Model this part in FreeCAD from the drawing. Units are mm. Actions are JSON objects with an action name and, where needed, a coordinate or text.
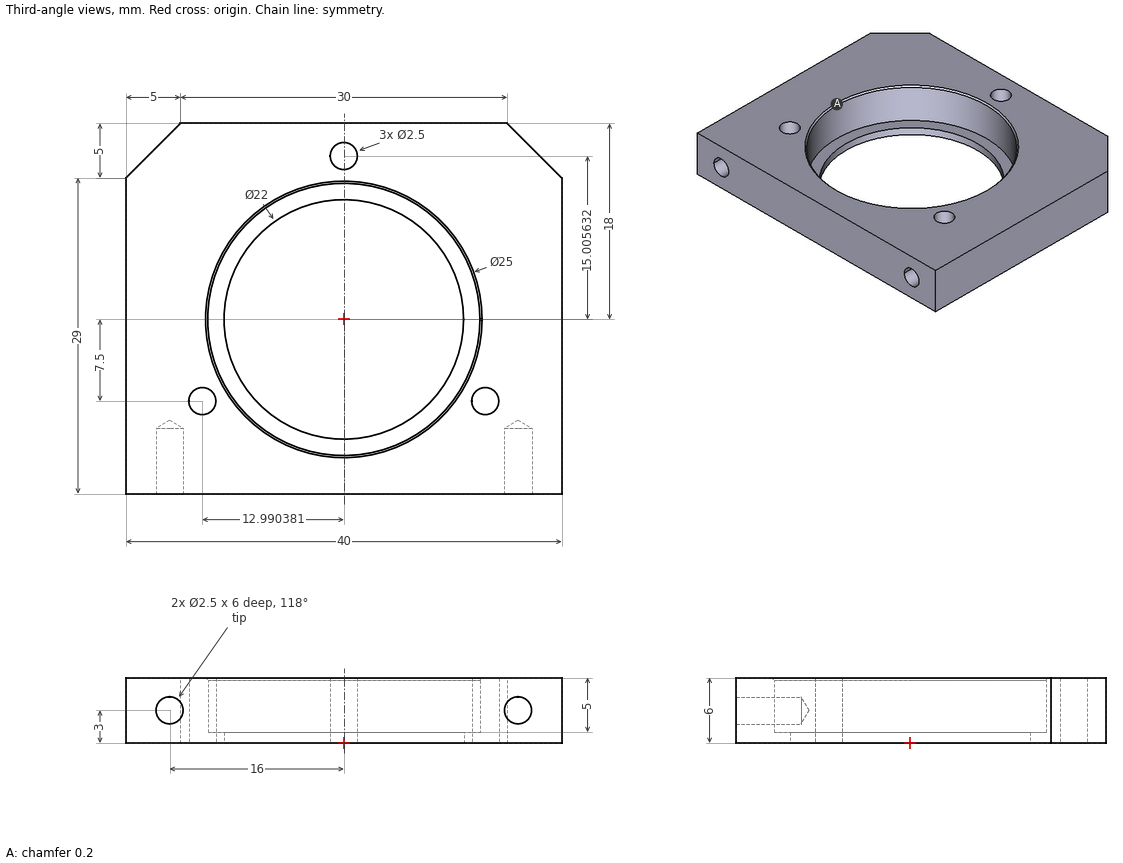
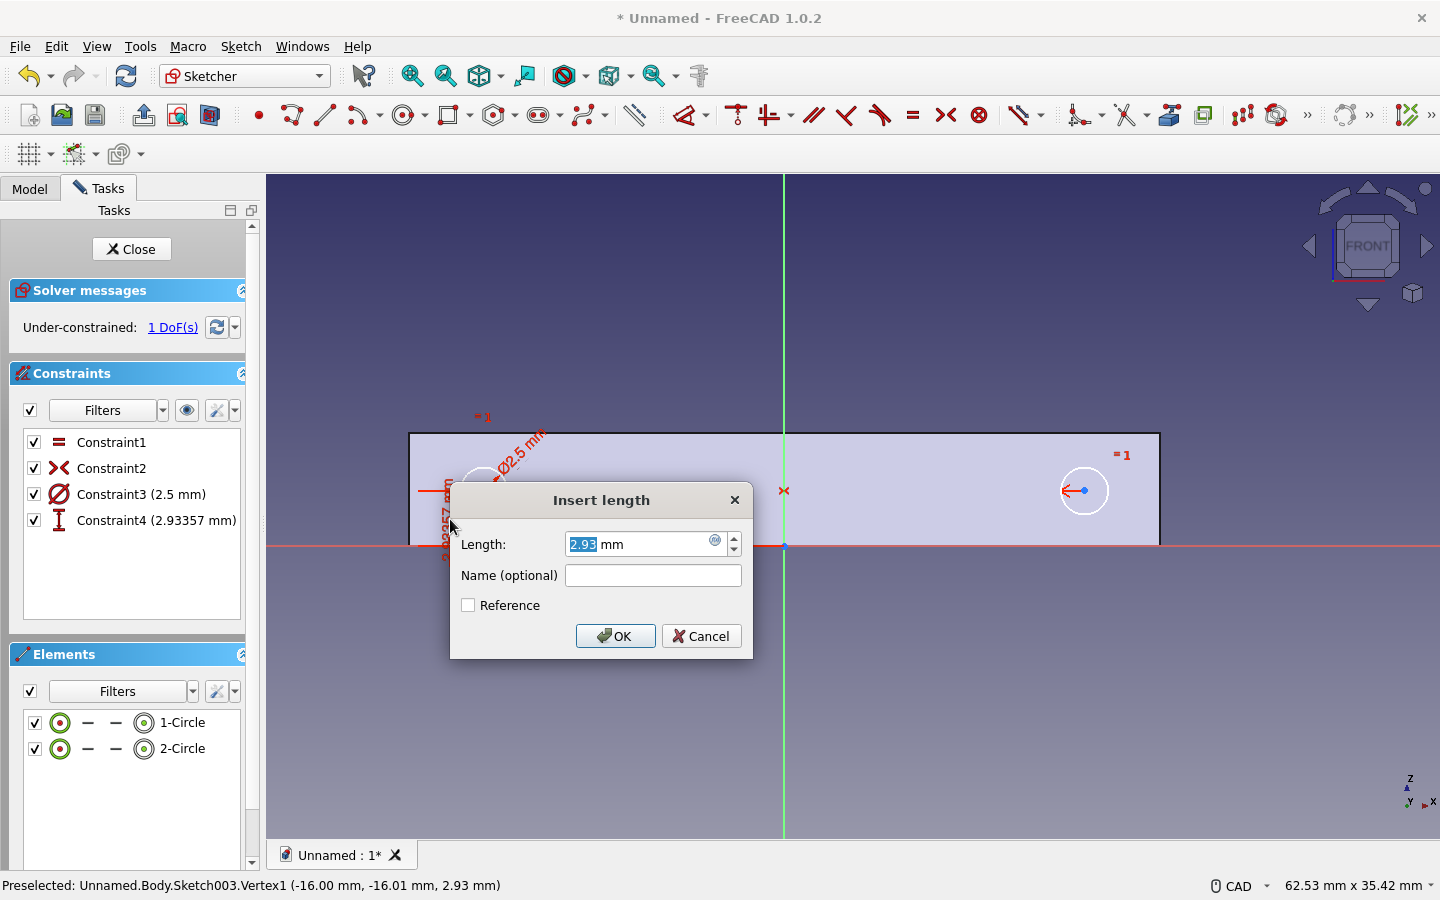
{"action": "type", "text": "3"}
{"action": "key", "text": "Return"}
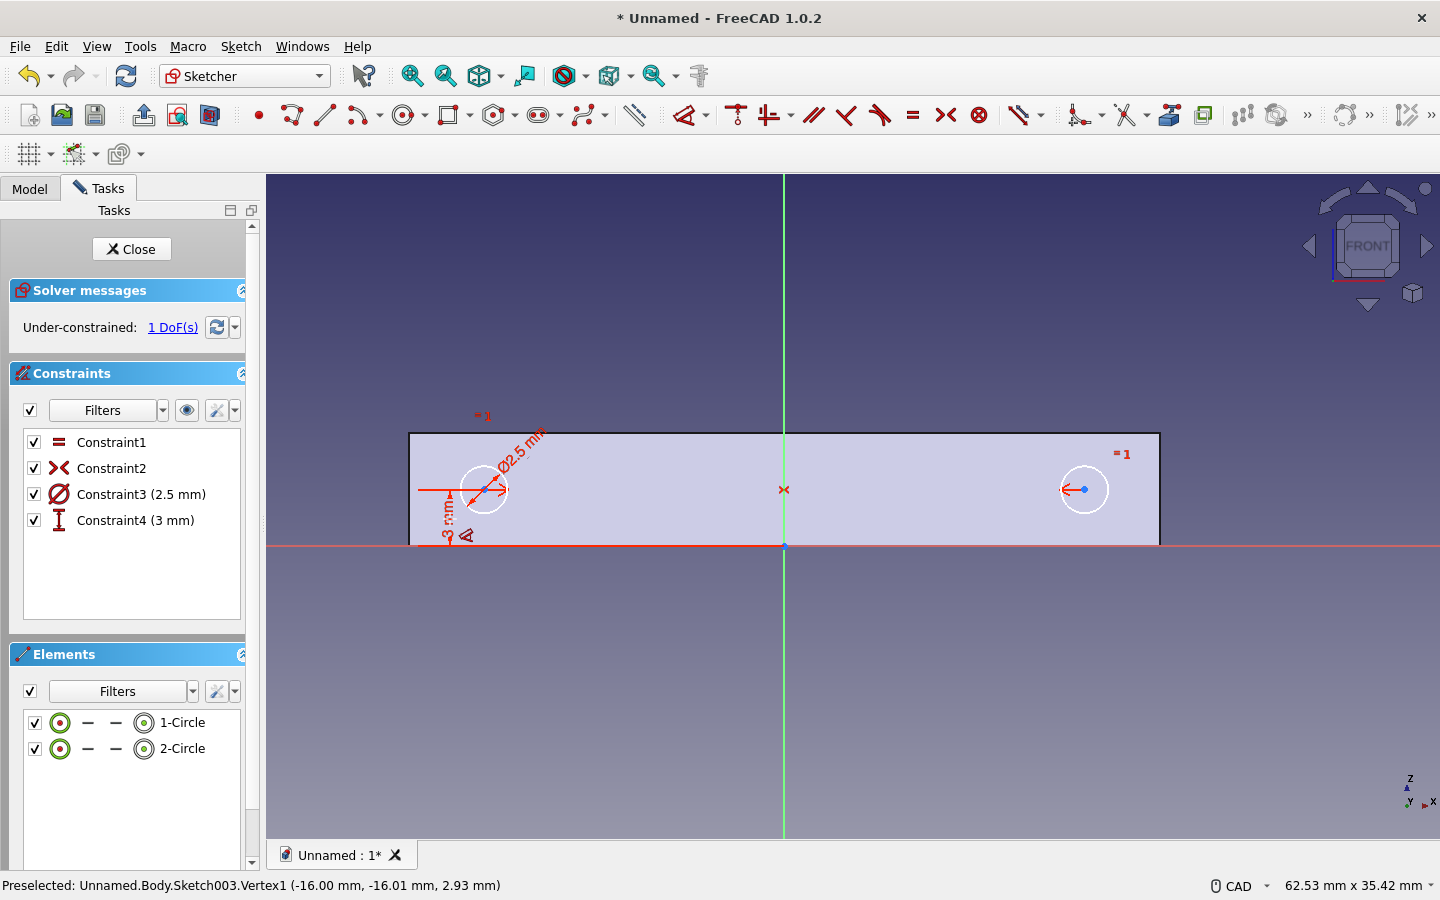
{"action": "left_click", "coordinate": [484, 490]}
{"action": "left_click", "coordinate": [634, 580]}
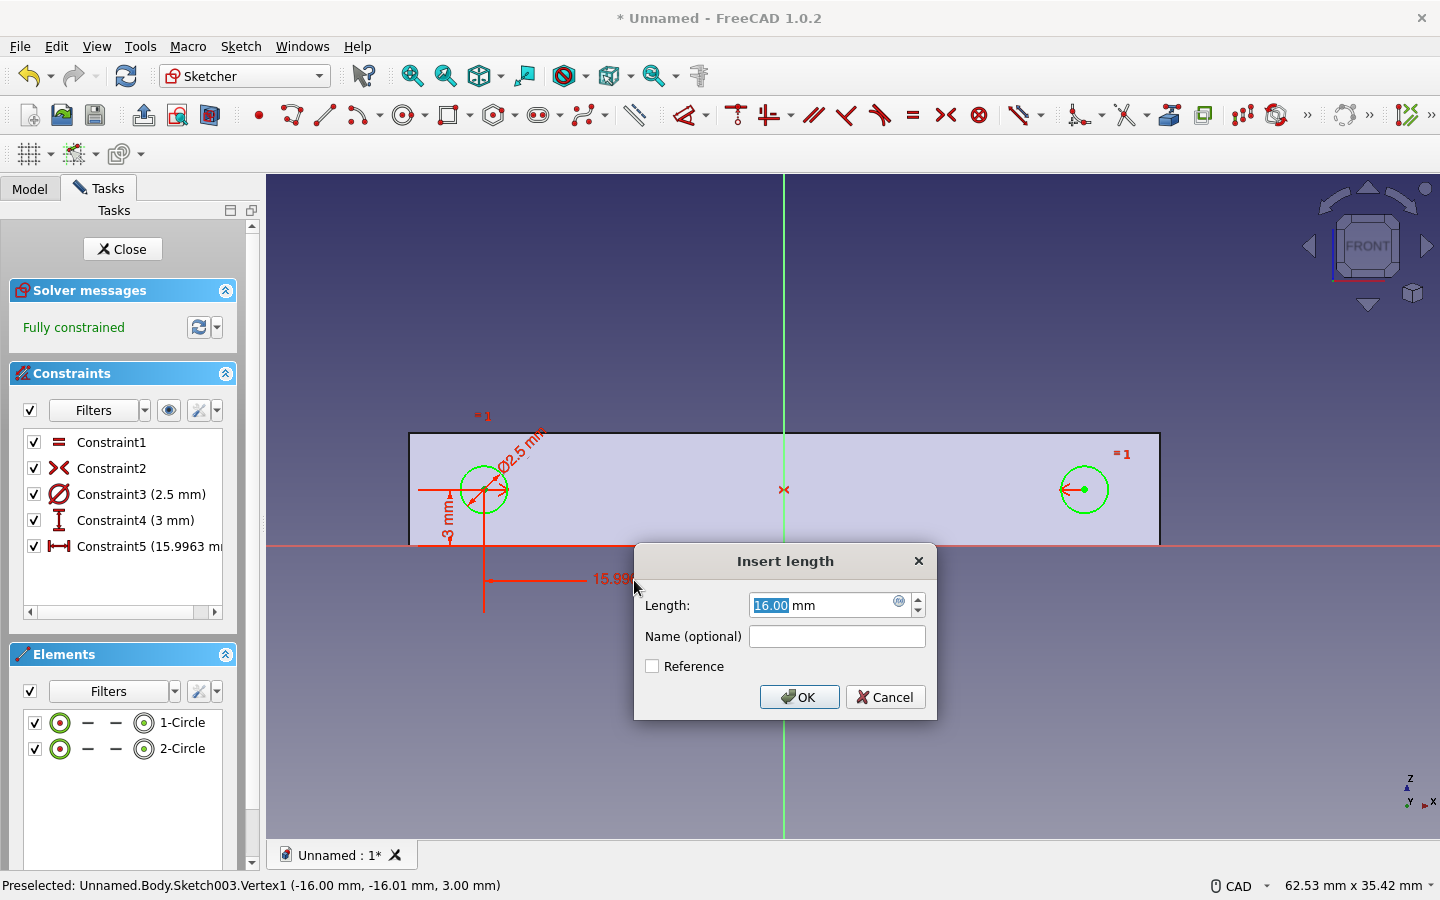
{"action": "type", "text": "16"}
{"action": "key", "text": "Return"}
{"action": "key", "text": "Escape"}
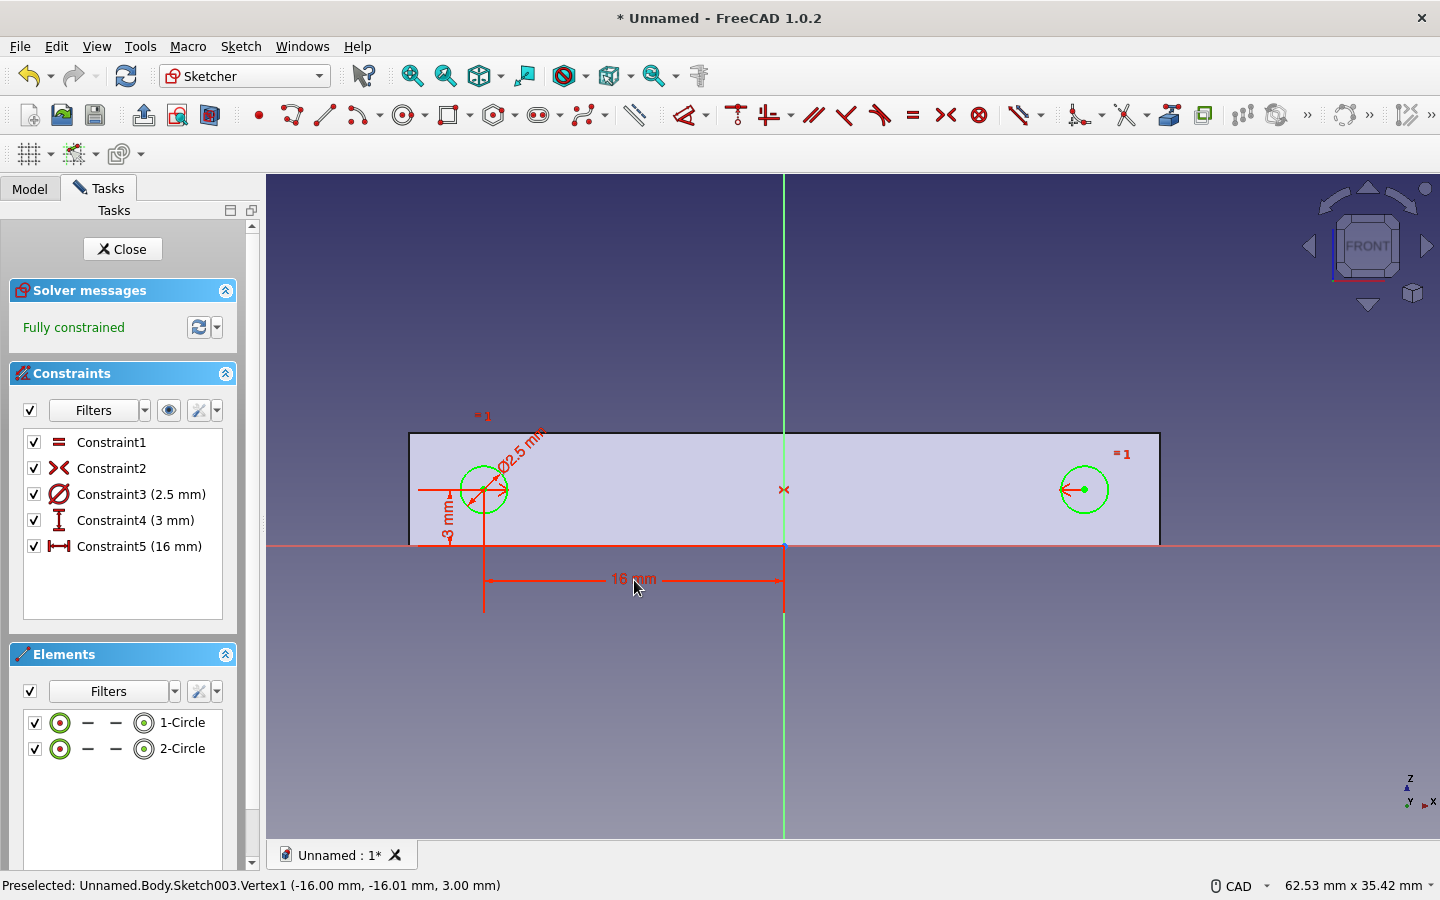
{"action": "left_click", "coordinate": [123, 249]}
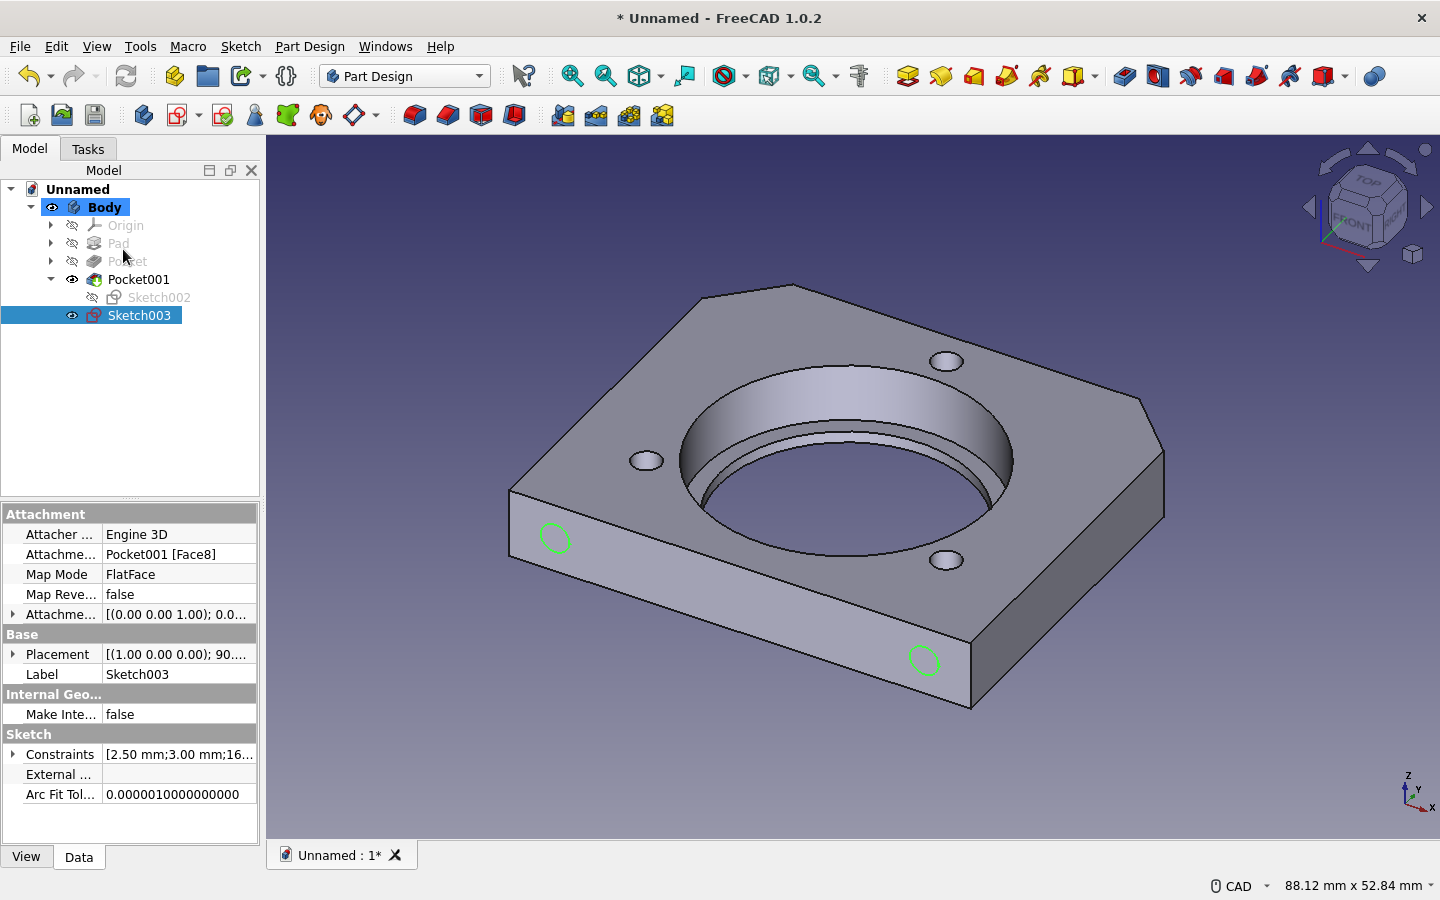
{"action": "left_click", "coordinate": [1158, 76]}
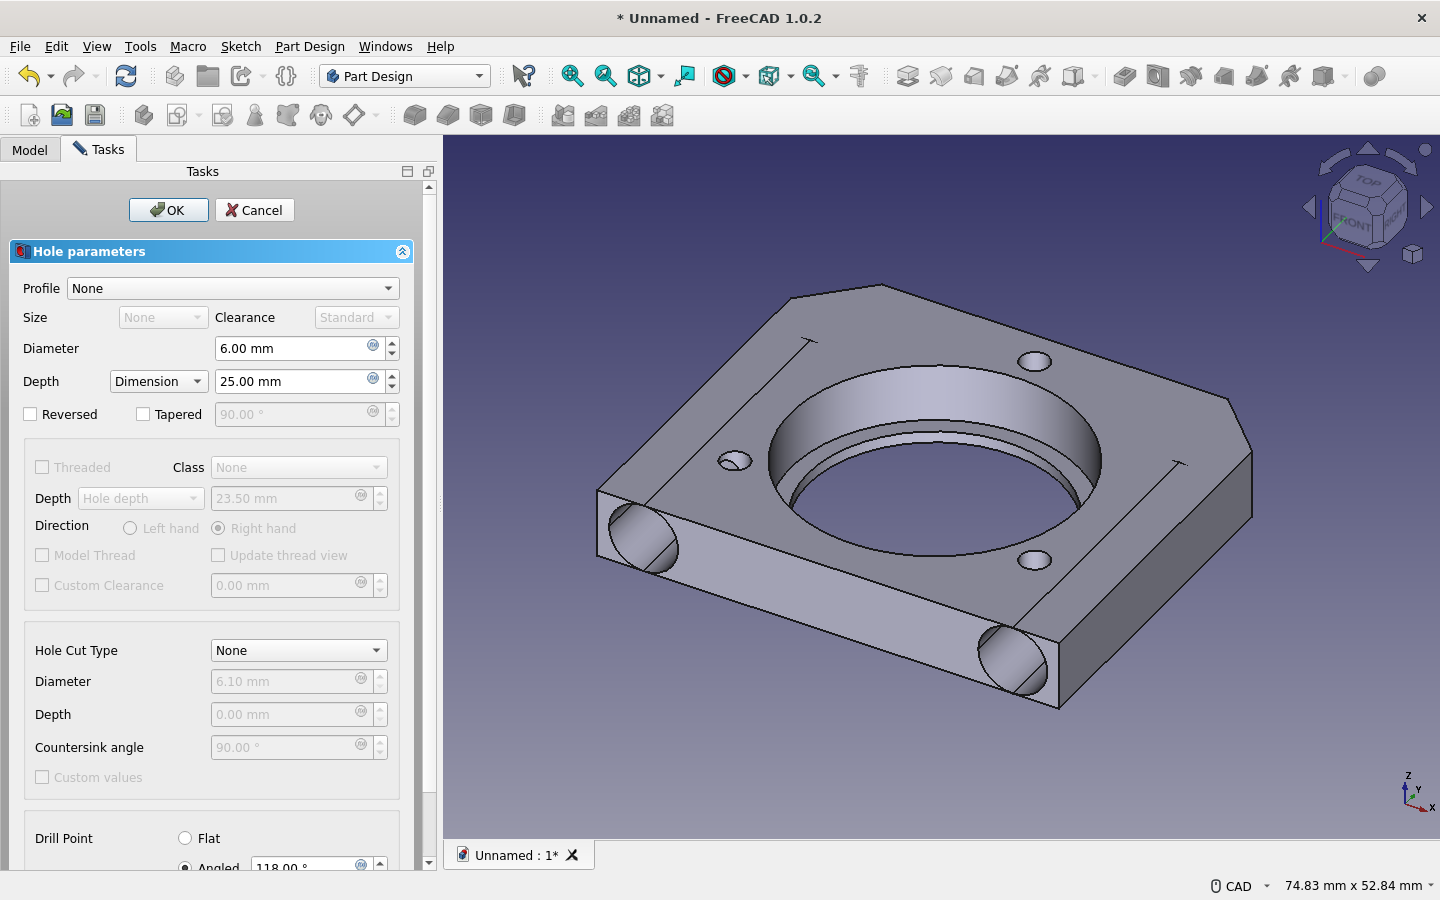
{"action": "triple_click", "coordinate": [300, 348]}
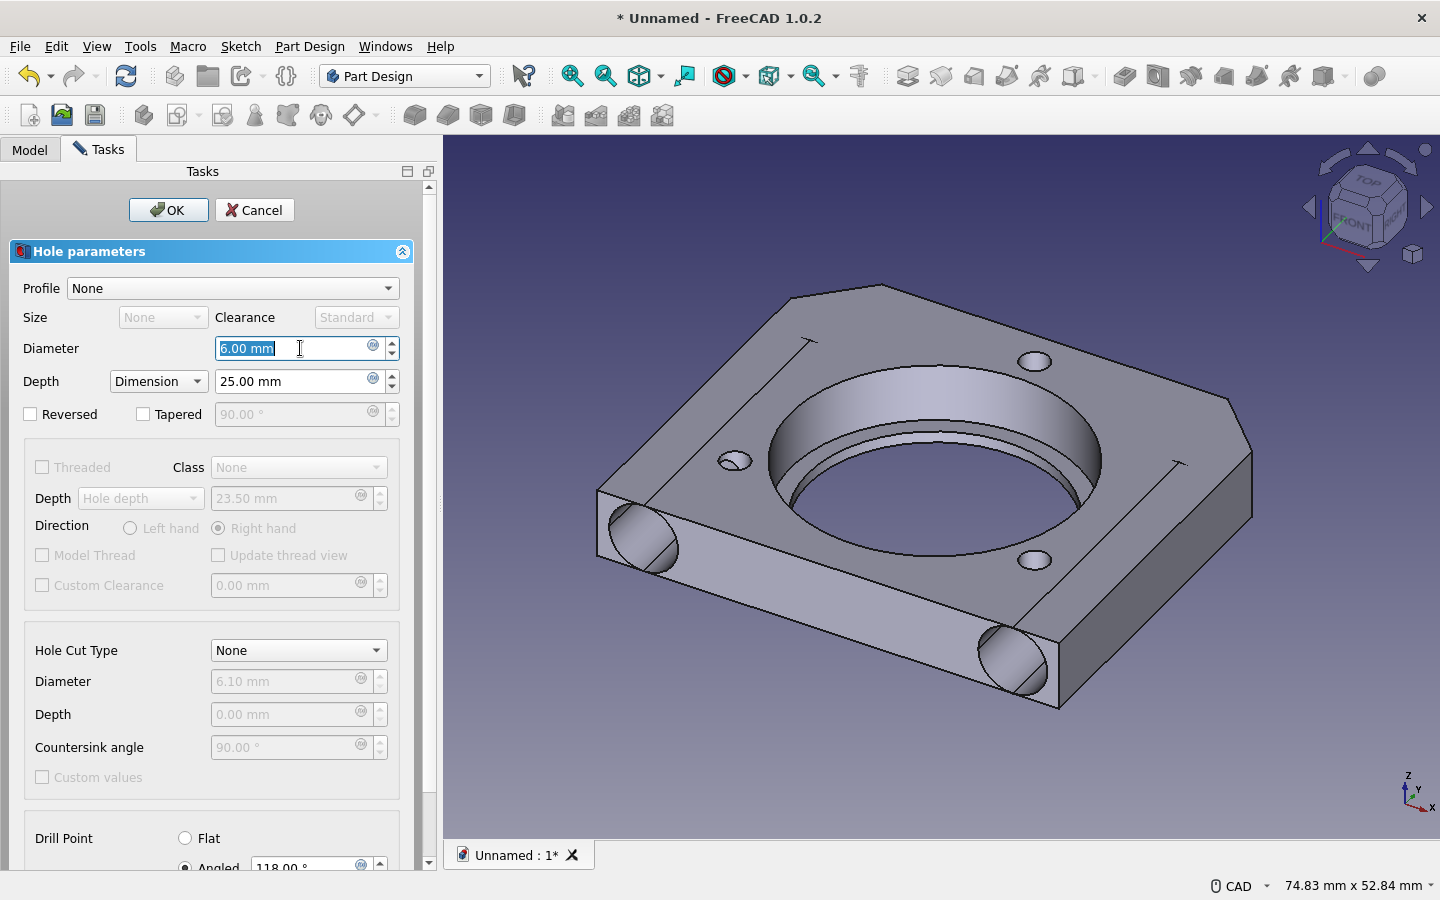
{"action": "type", "text": "2.5"}
{"action": "key", "text": "Tab"}